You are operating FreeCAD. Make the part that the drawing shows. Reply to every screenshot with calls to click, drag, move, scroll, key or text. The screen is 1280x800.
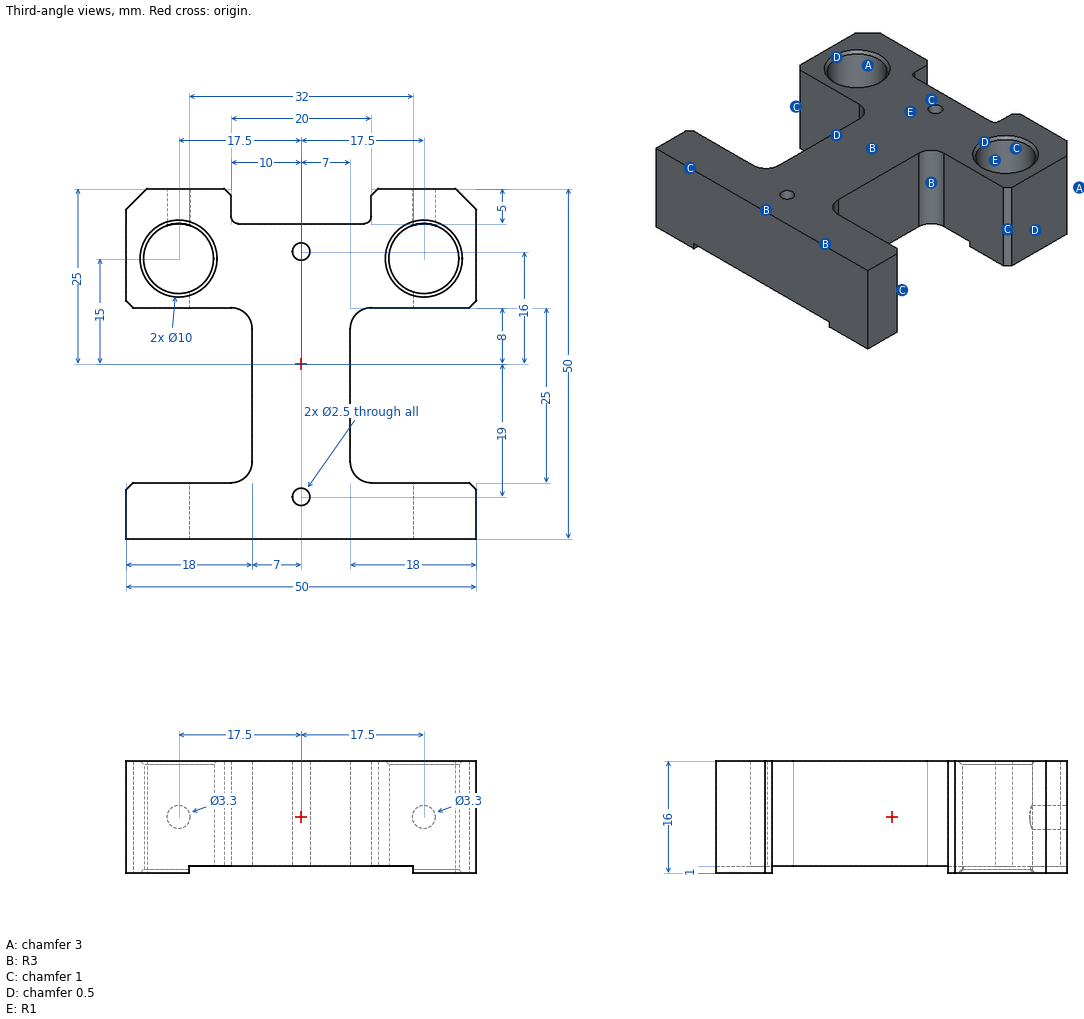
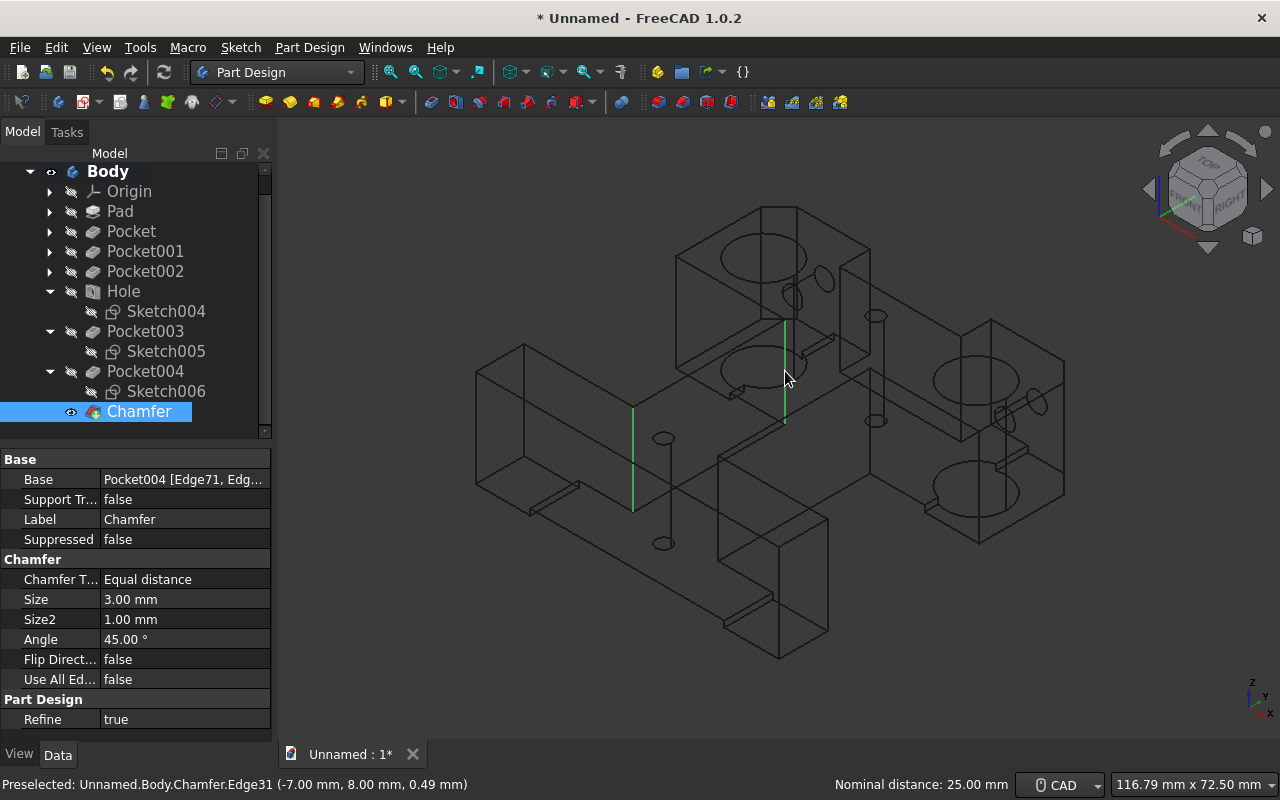
click(718, 497, ctrl)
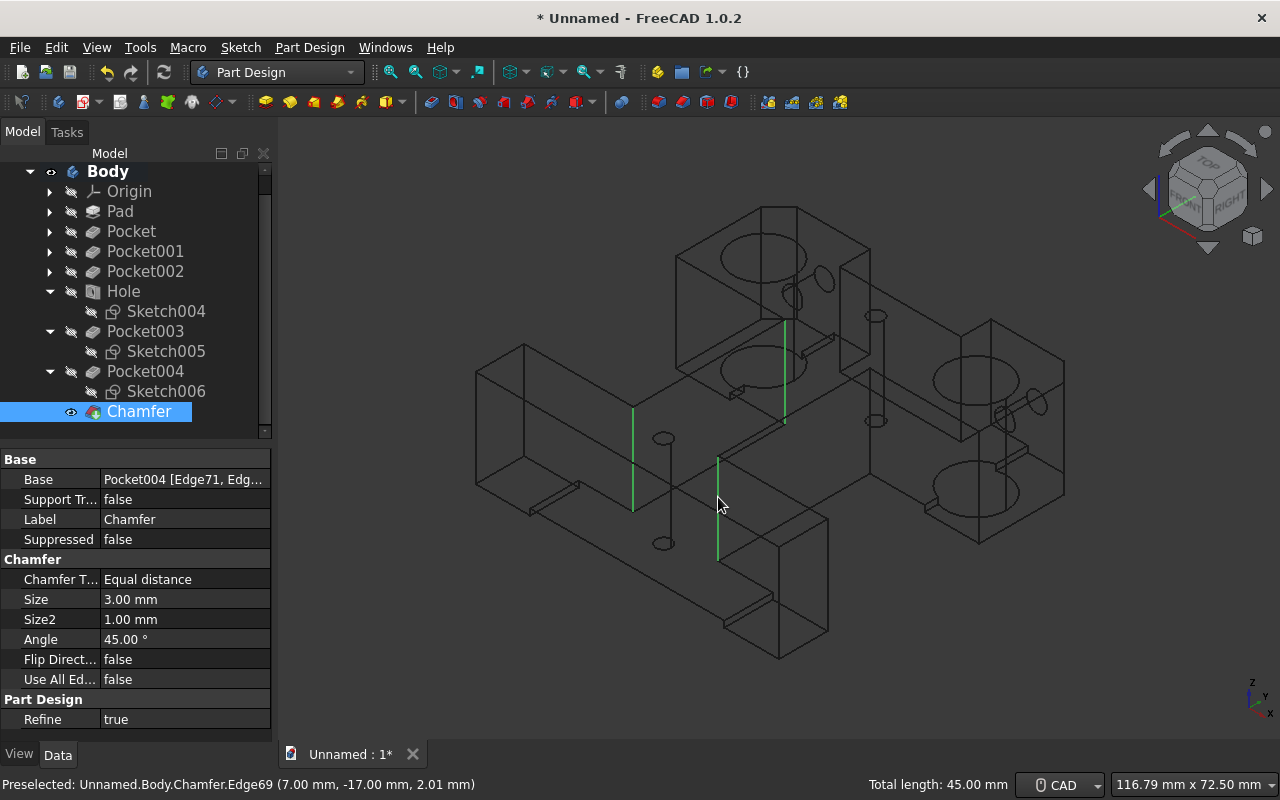
click(870, 420, ctrl)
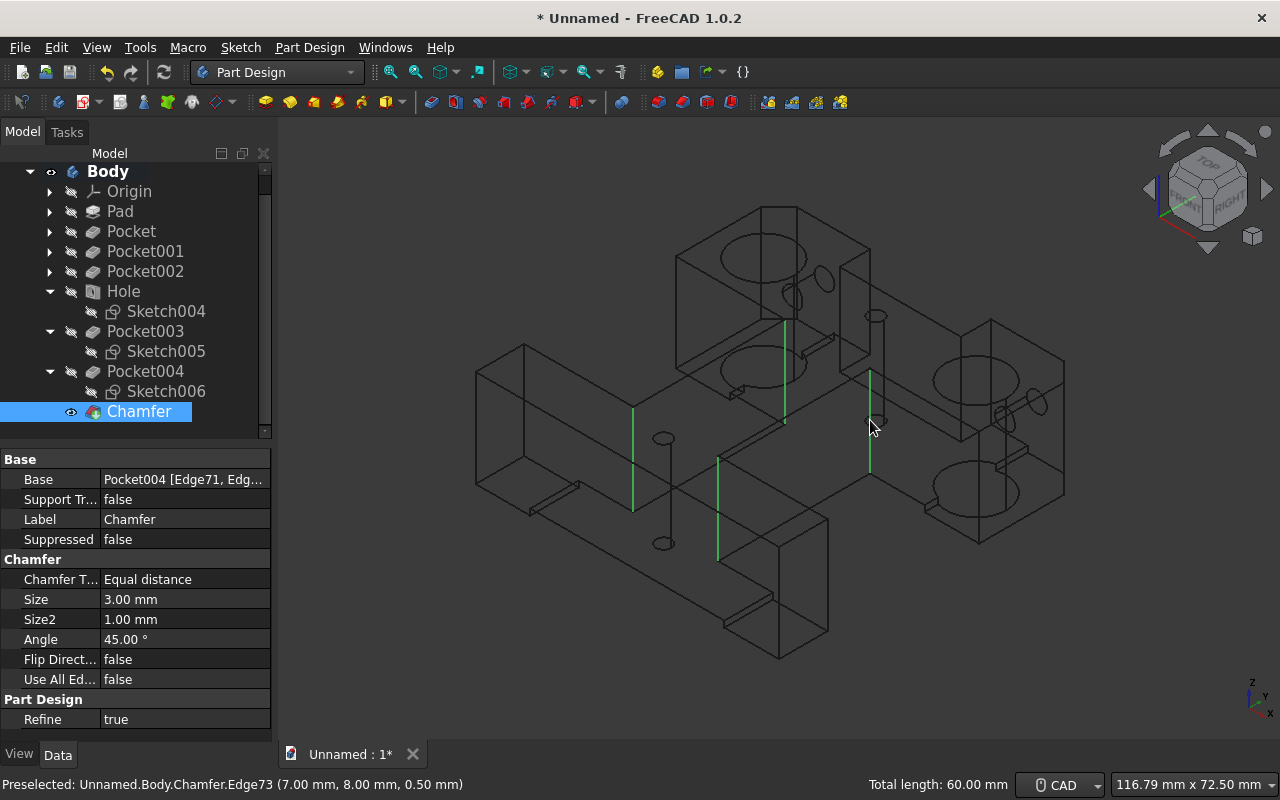
key(v)
key(1)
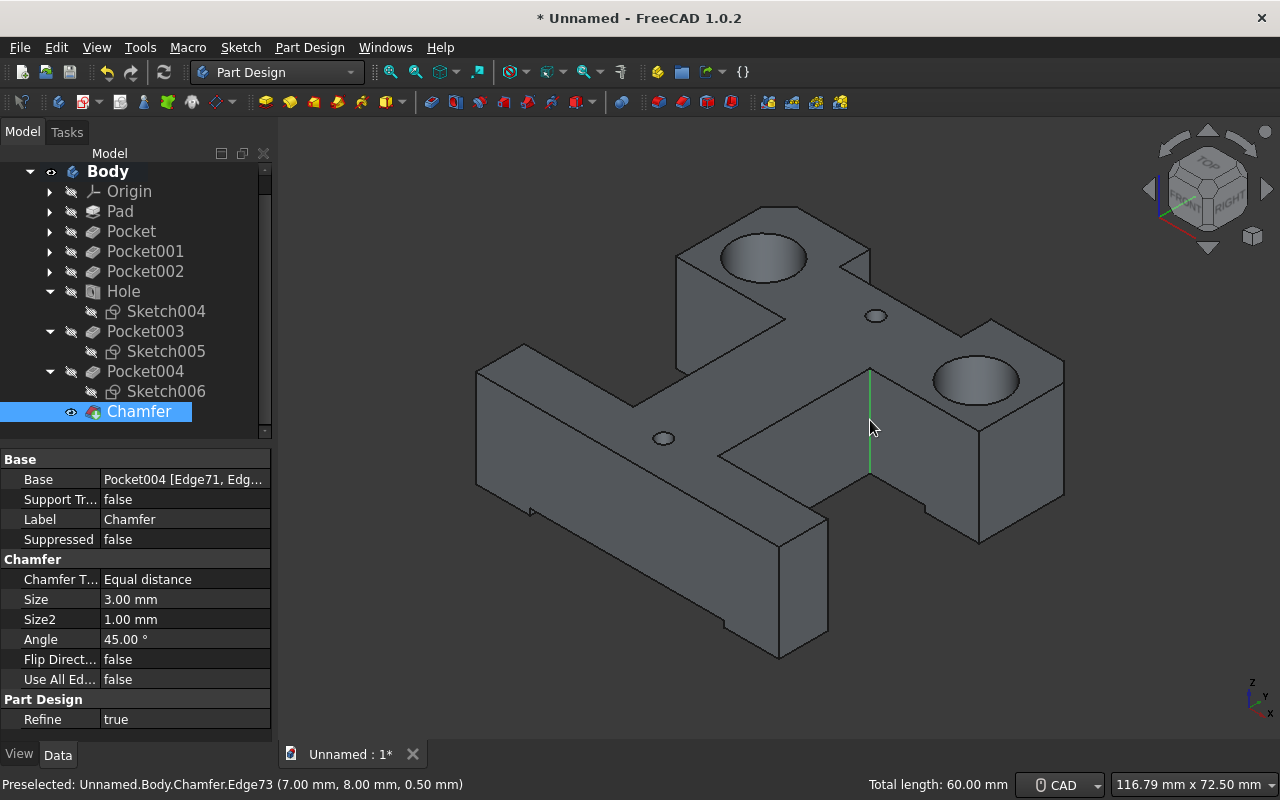
click(660, 102)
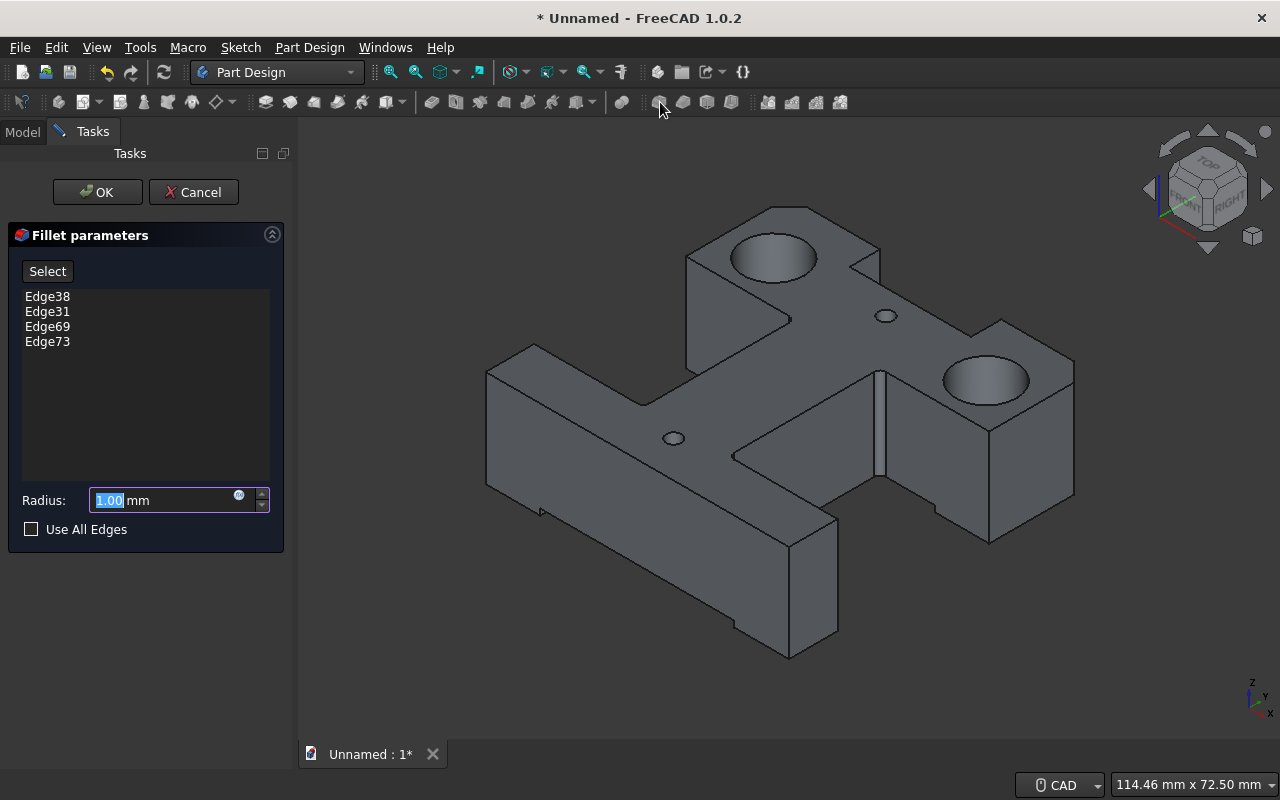
text(3)
key(Tab)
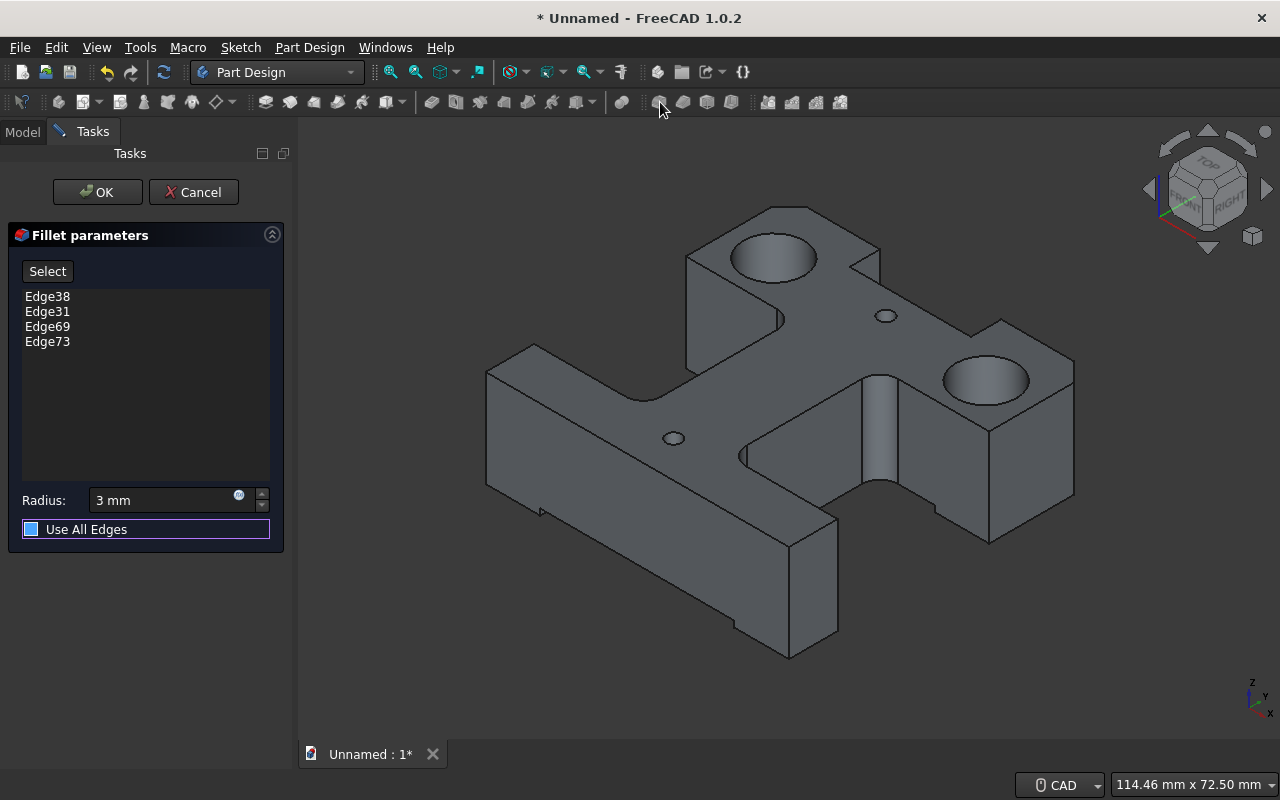
click(98, 192)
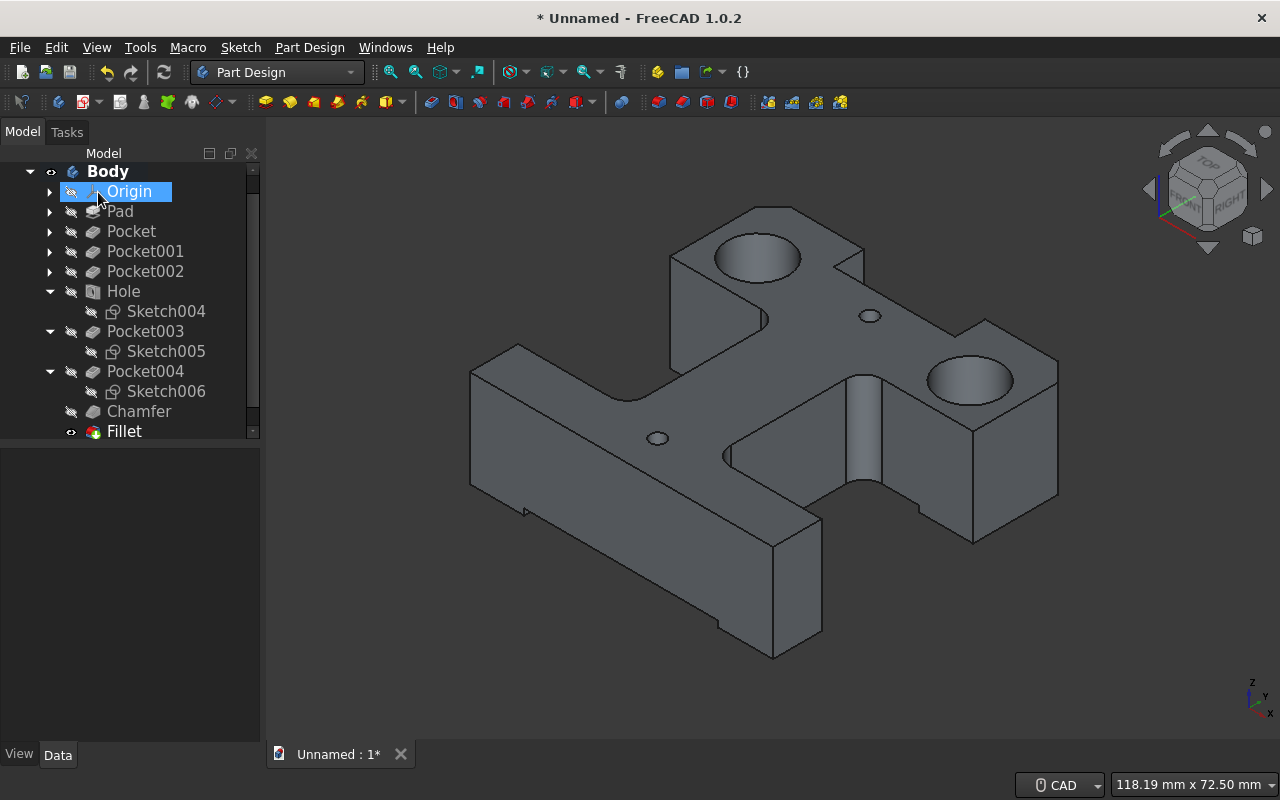
click(973, 487)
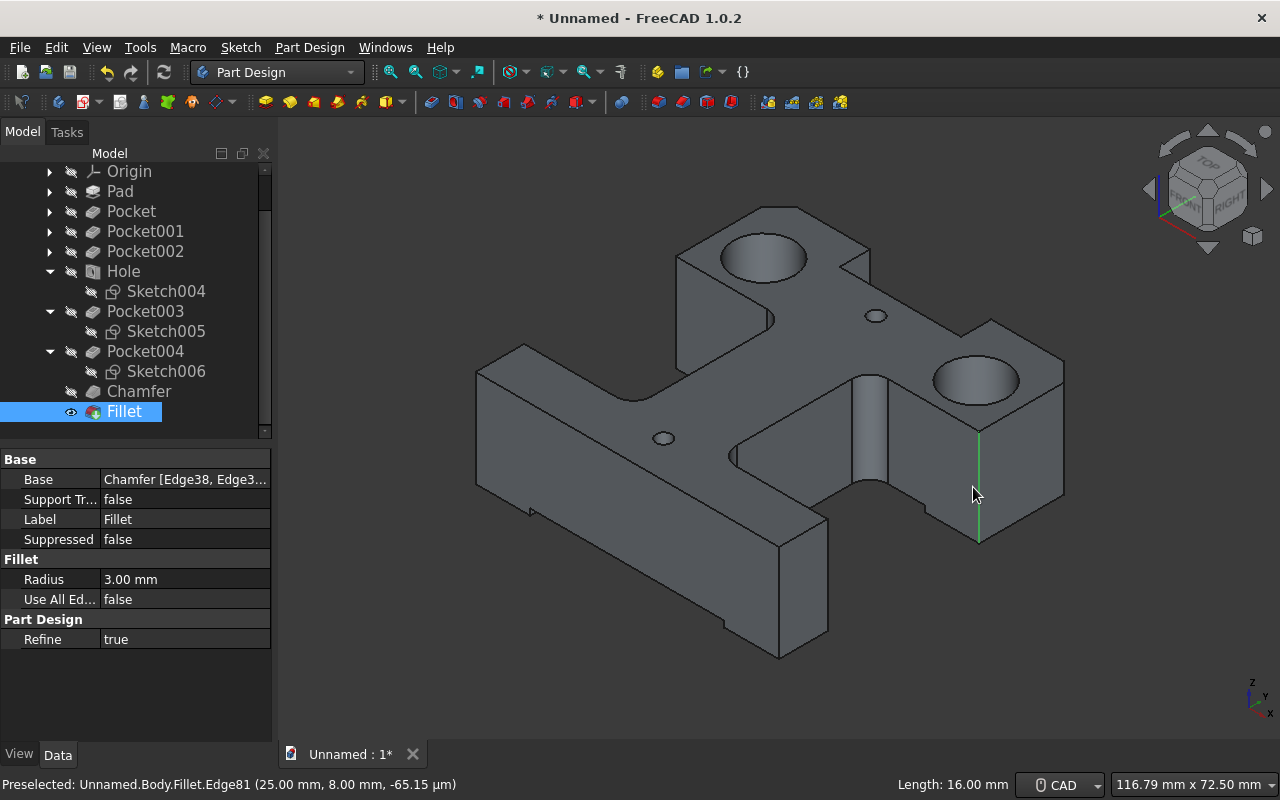
key(2)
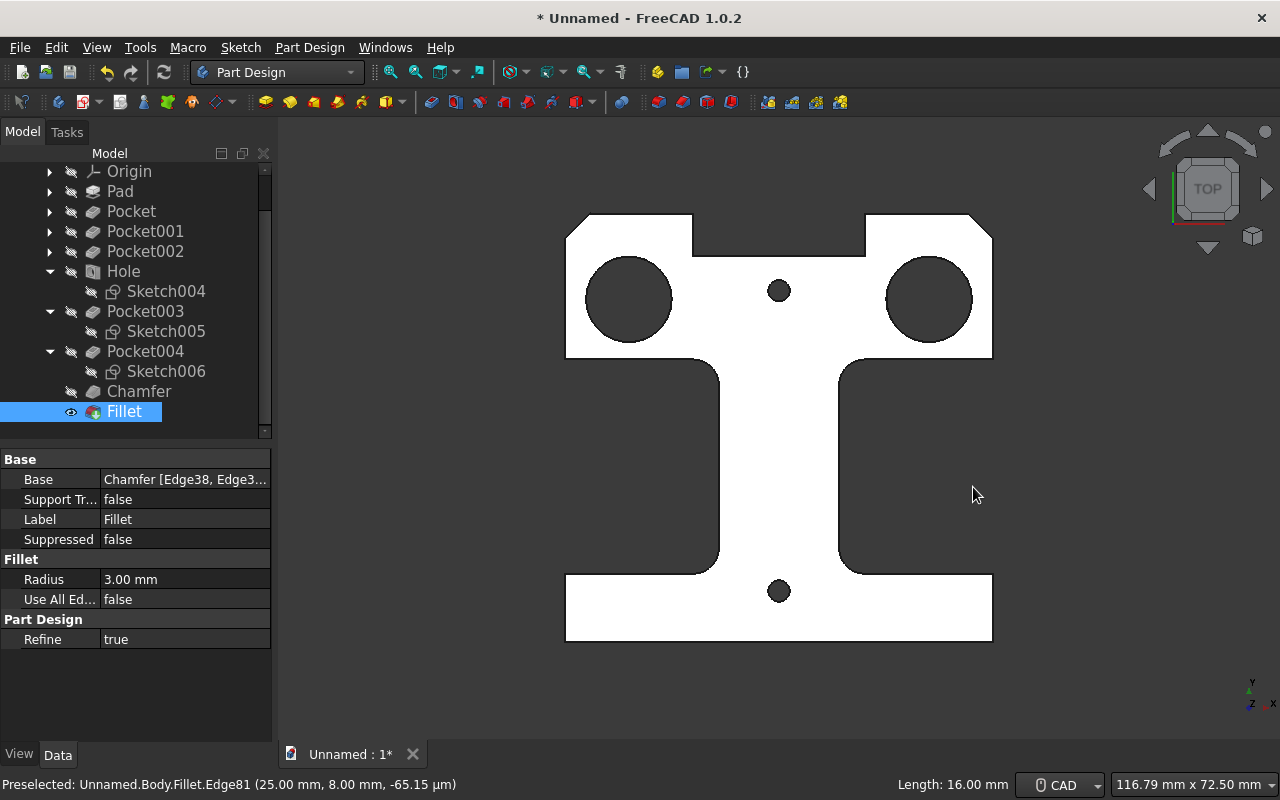
key(0)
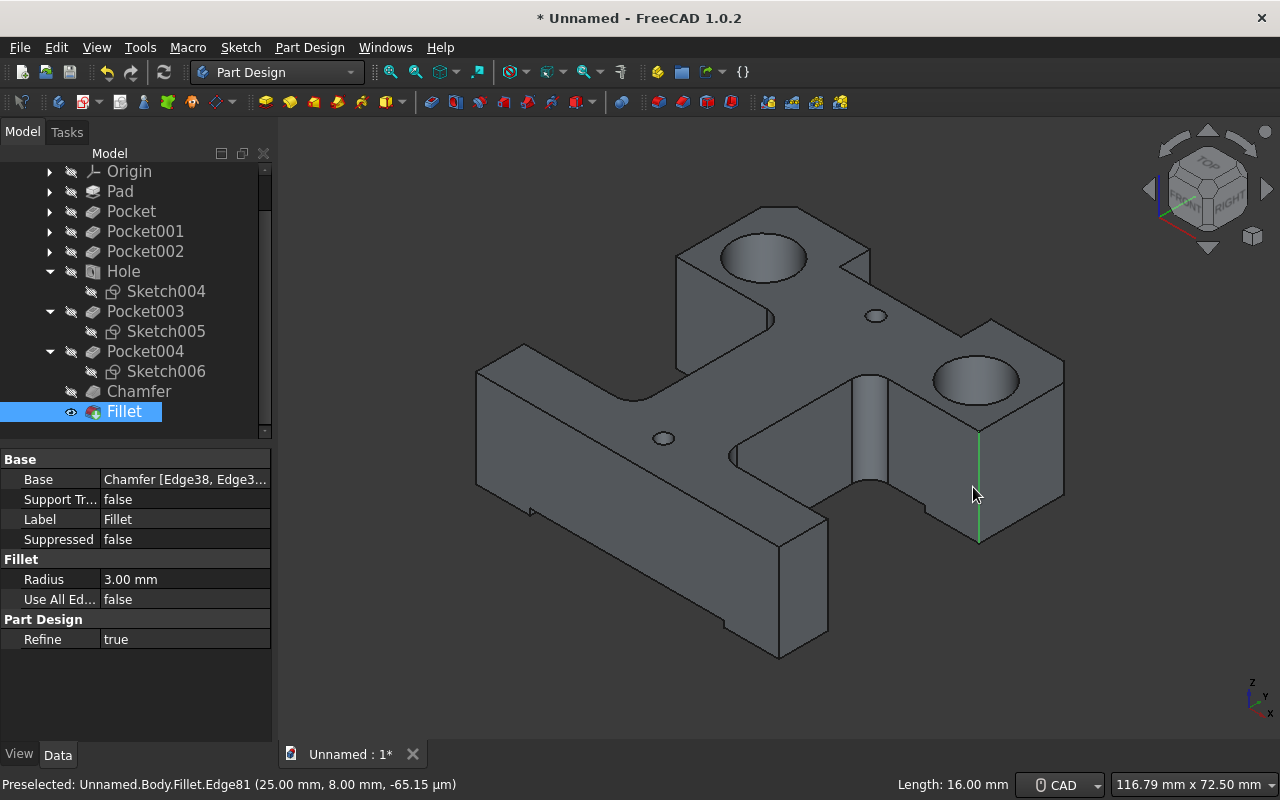
key(1)